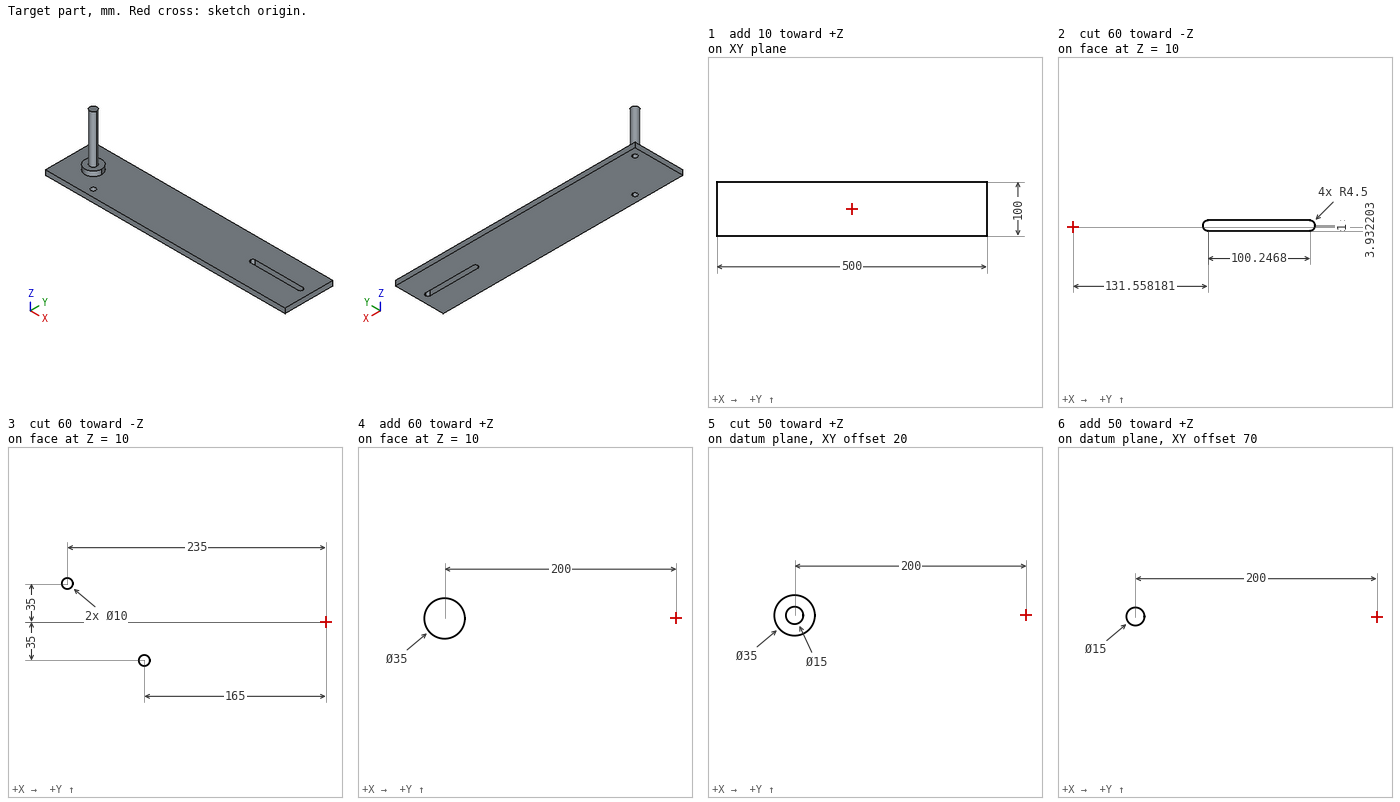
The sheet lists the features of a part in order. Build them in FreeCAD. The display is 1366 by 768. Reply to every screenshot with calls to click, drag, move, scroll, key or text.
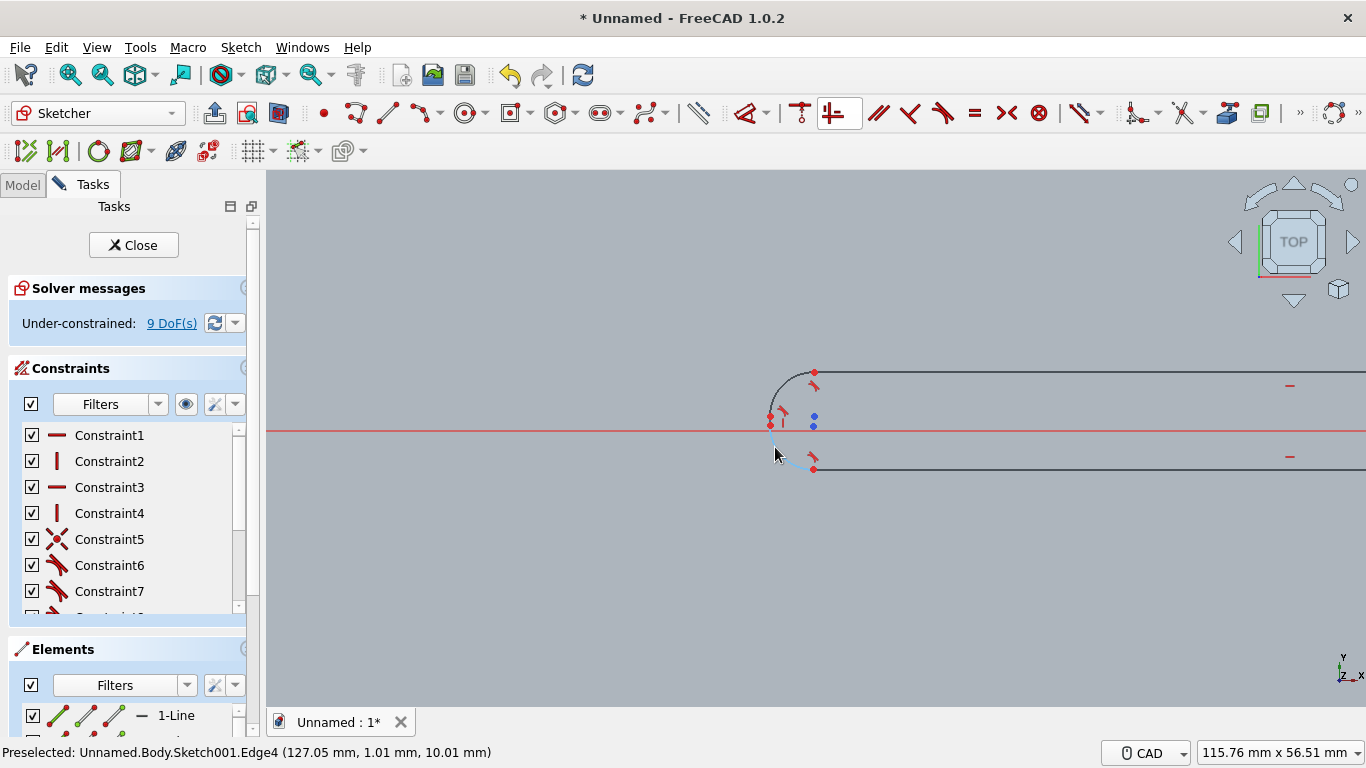
click(775, 446)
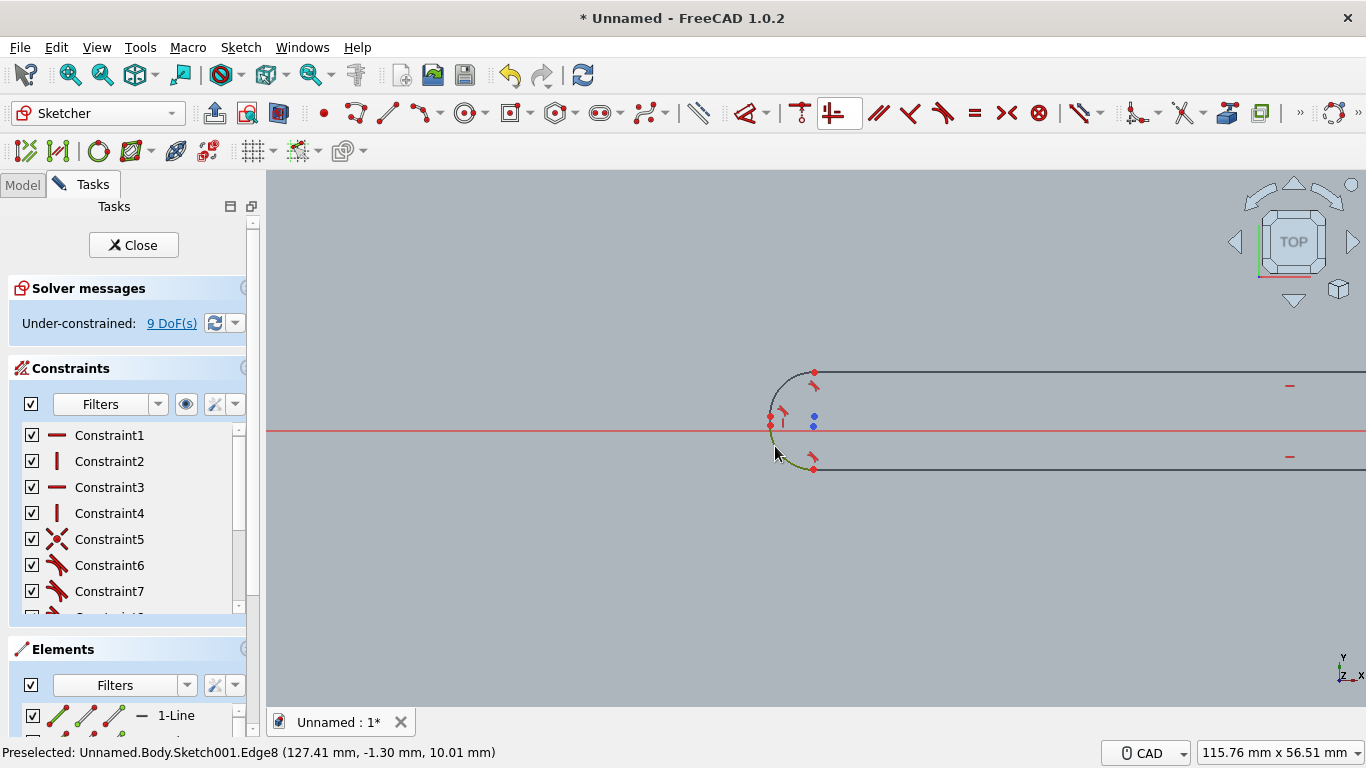
key(t)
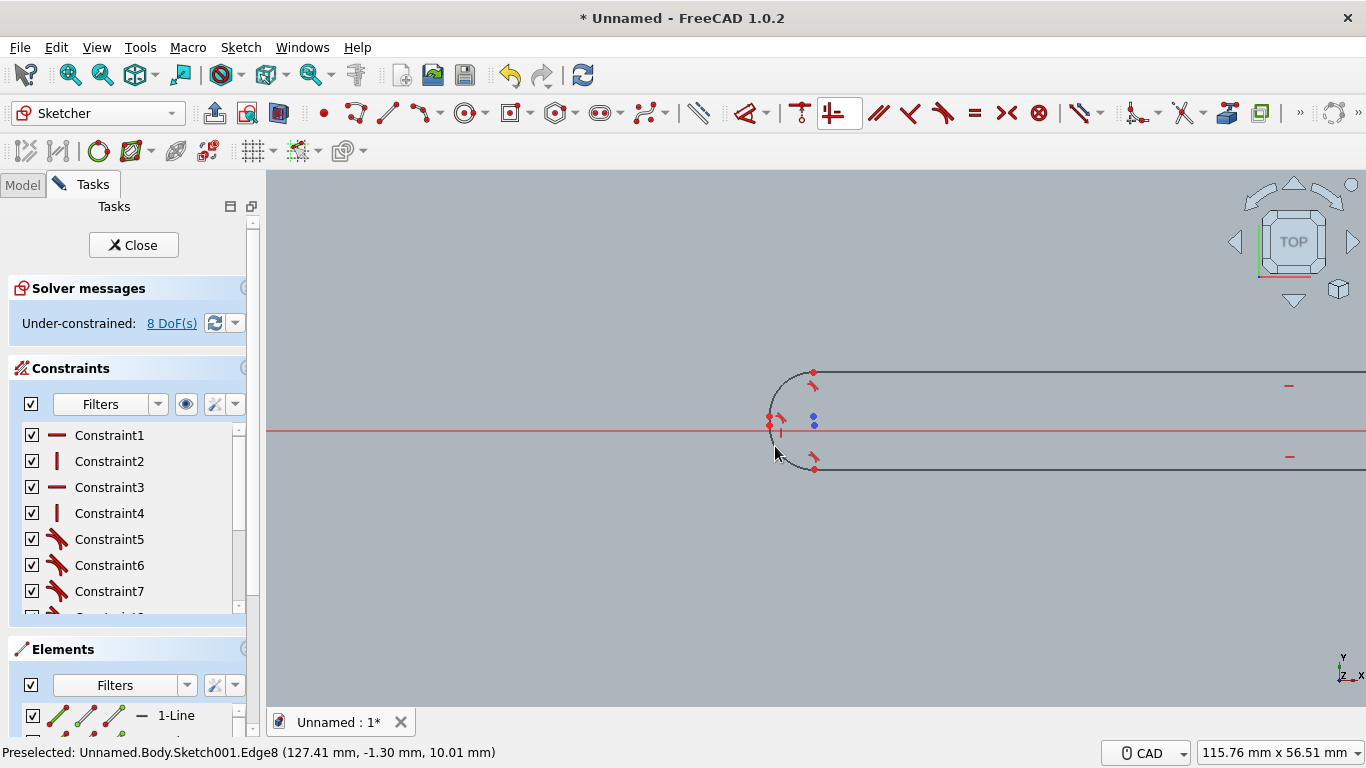
scroll(774, 446, down, 6)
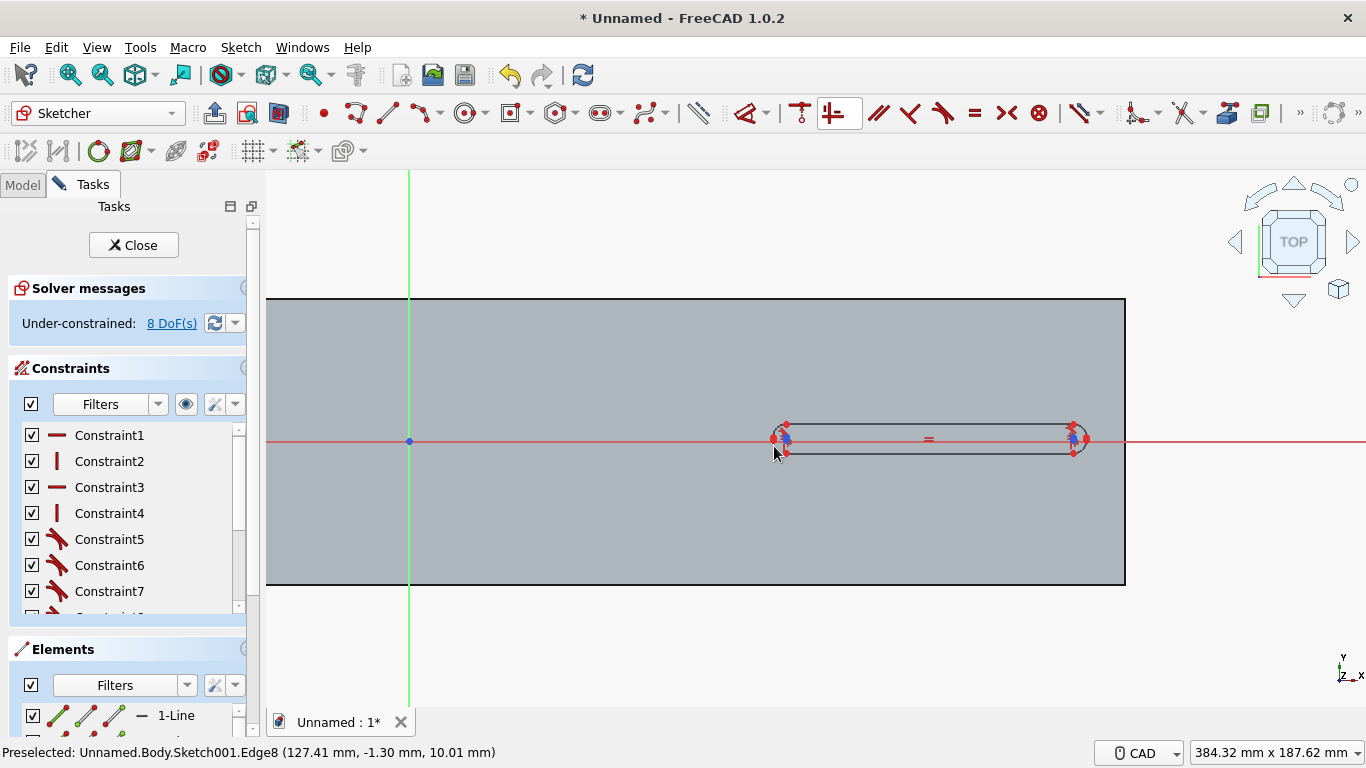
scroll(1079, 452, up, 4)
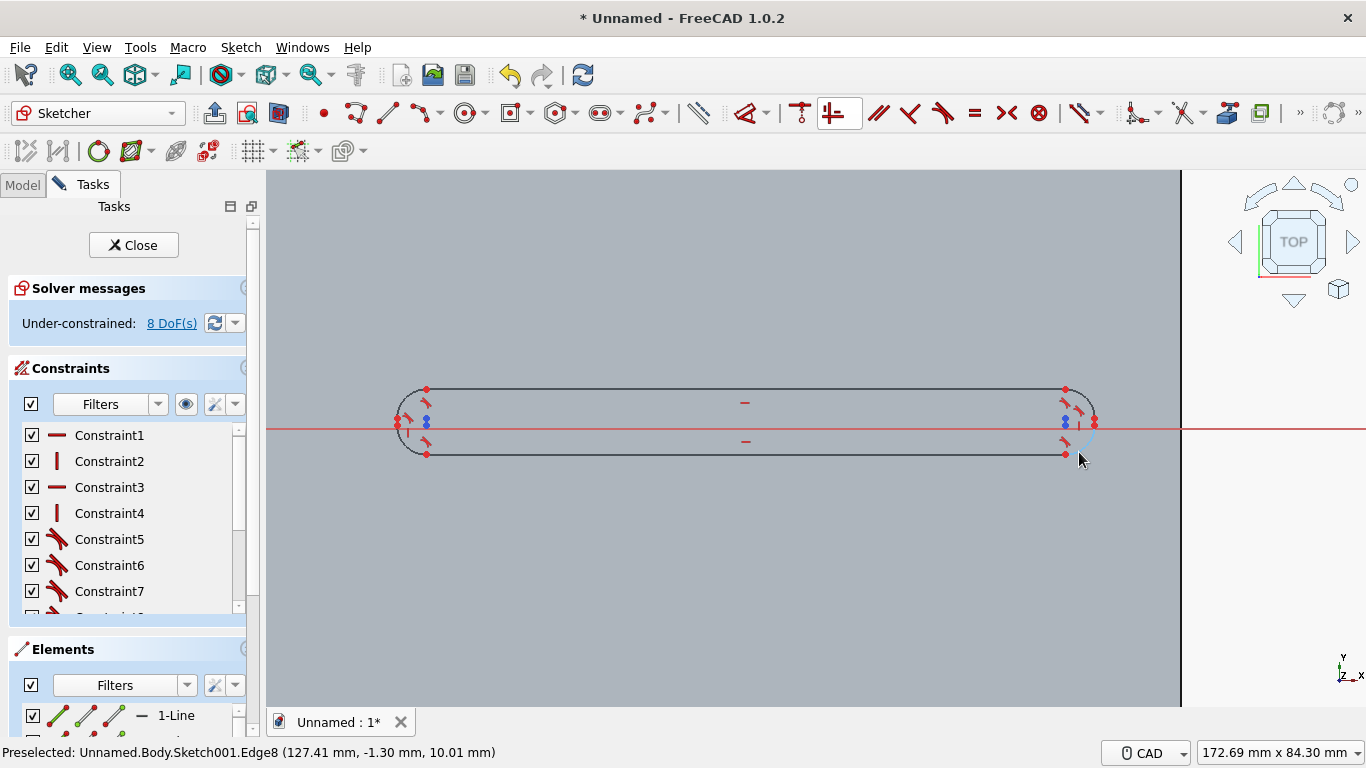
click(1079, 452)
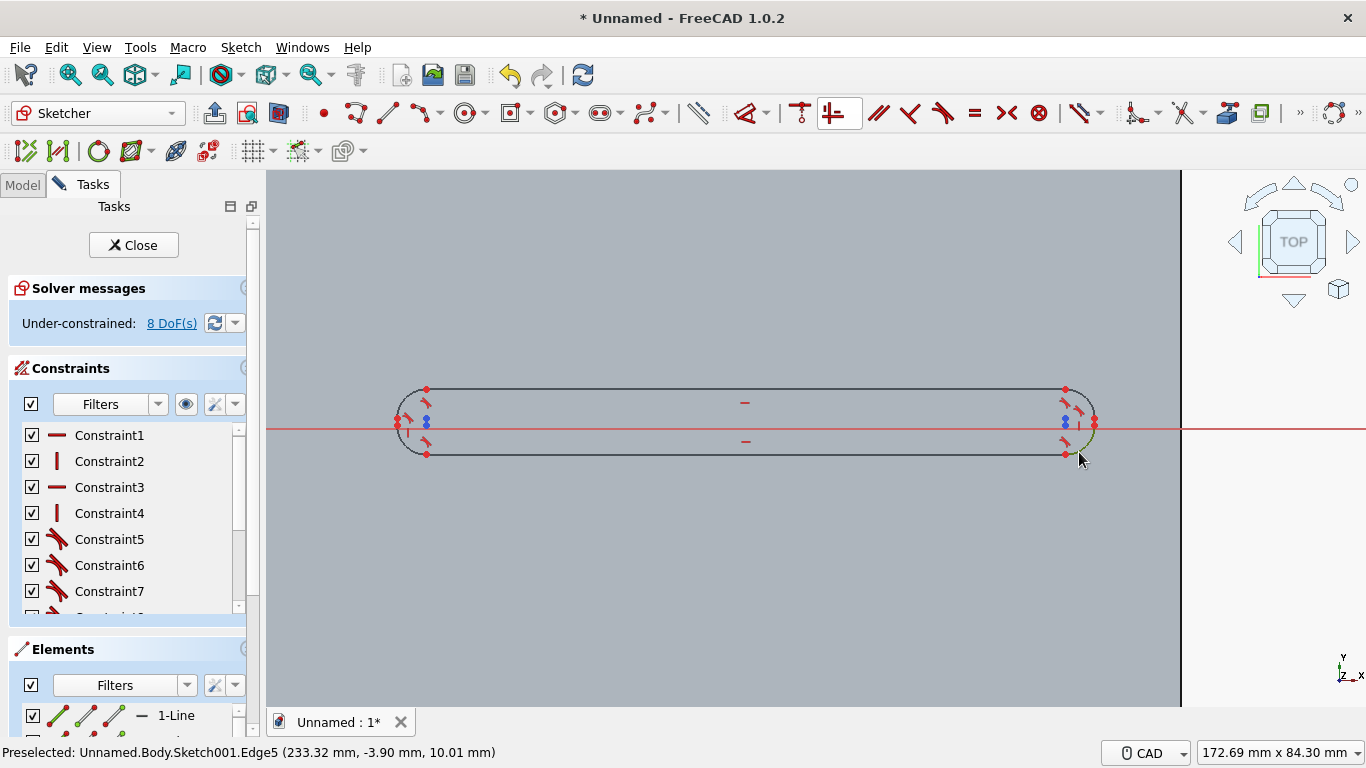
click(1092, 406)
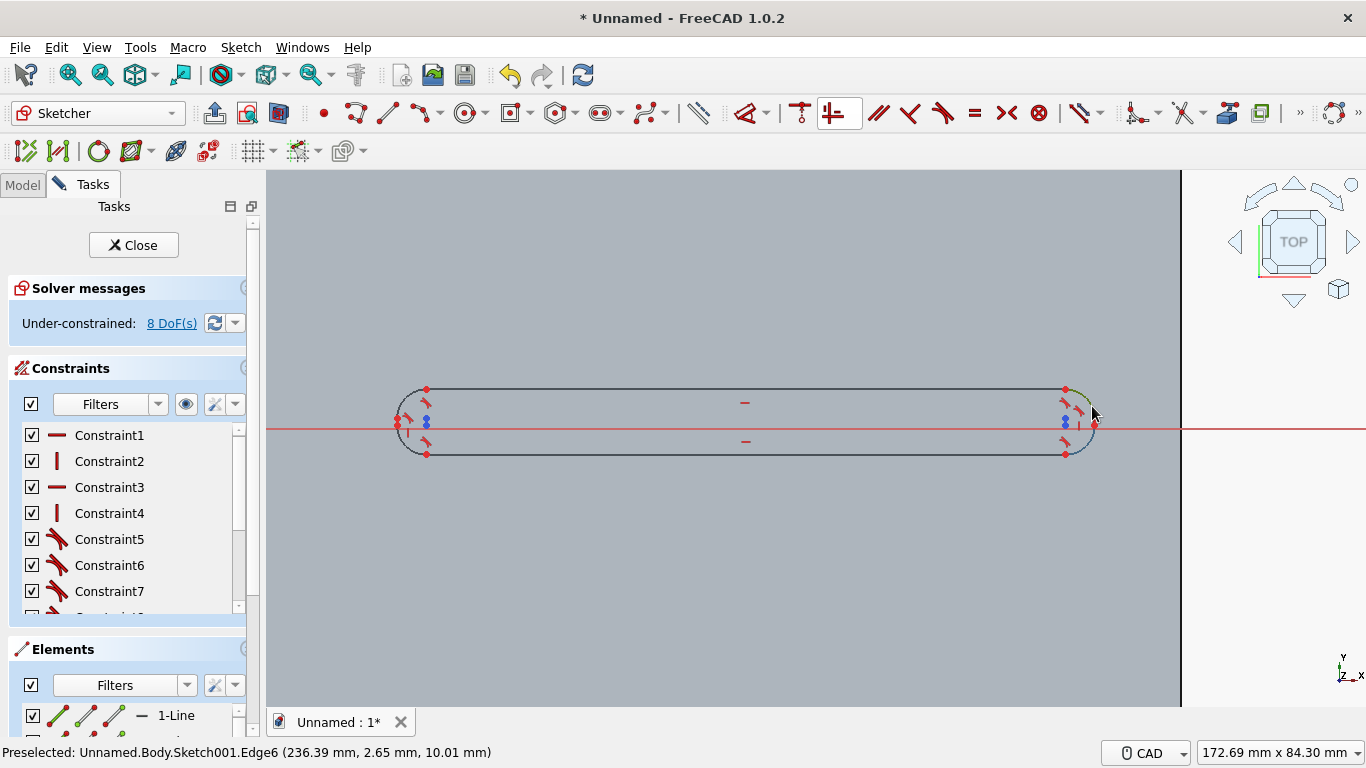
click(413, 393)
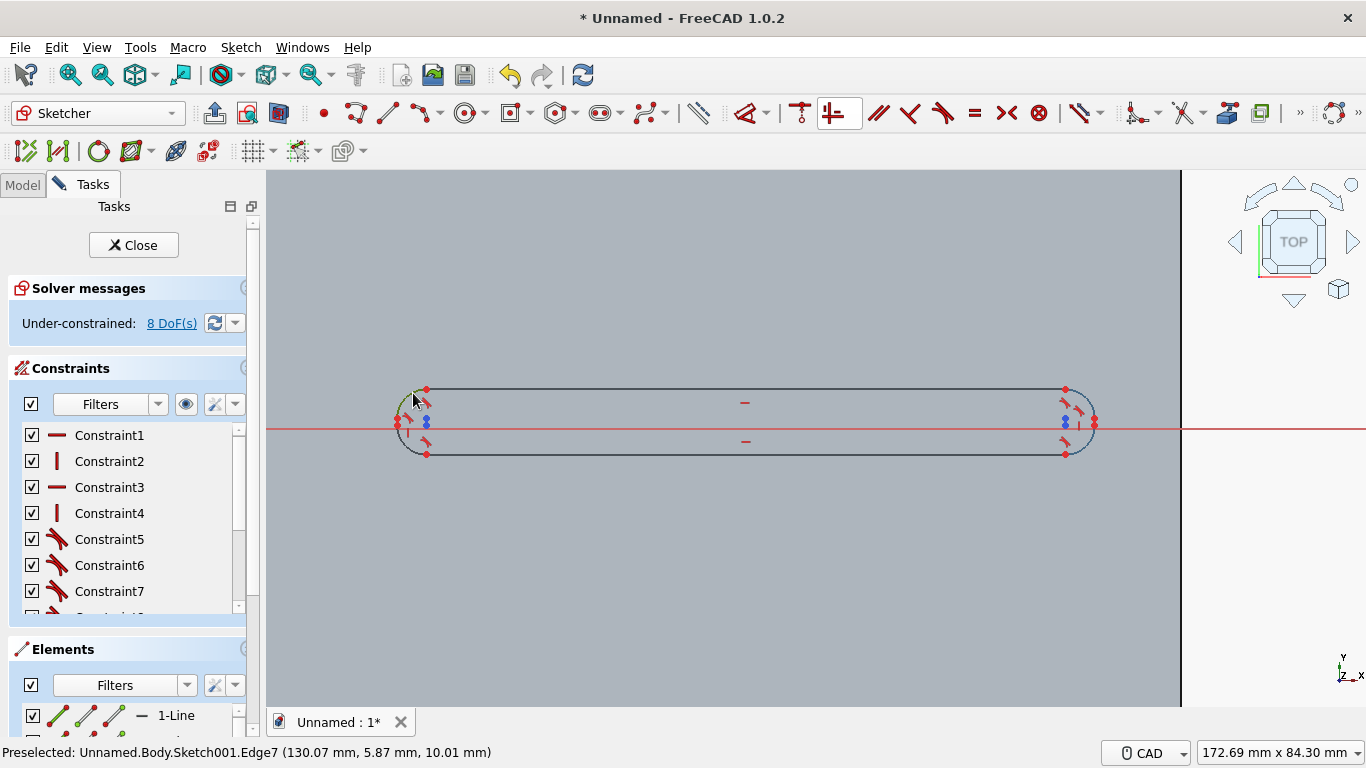
scroll(400, 439, up, 2)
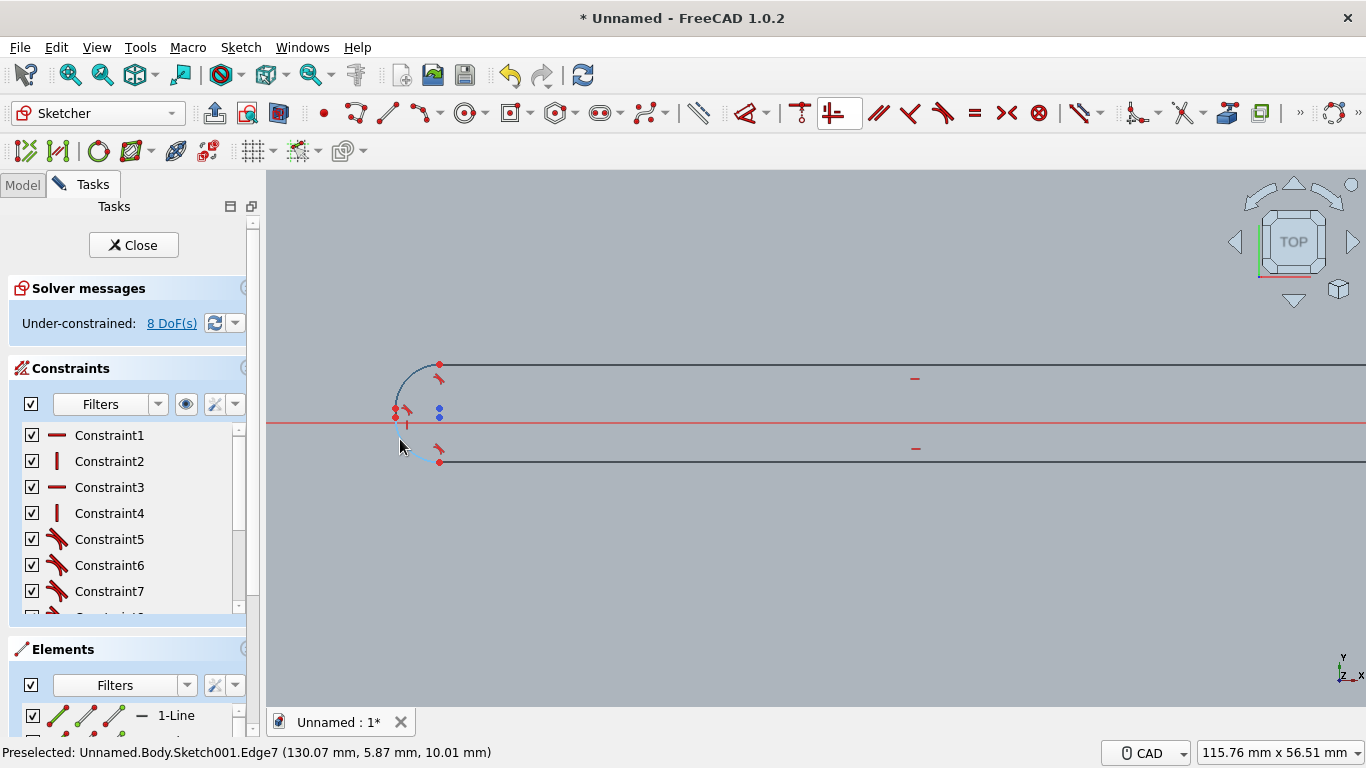
click(400, 438)